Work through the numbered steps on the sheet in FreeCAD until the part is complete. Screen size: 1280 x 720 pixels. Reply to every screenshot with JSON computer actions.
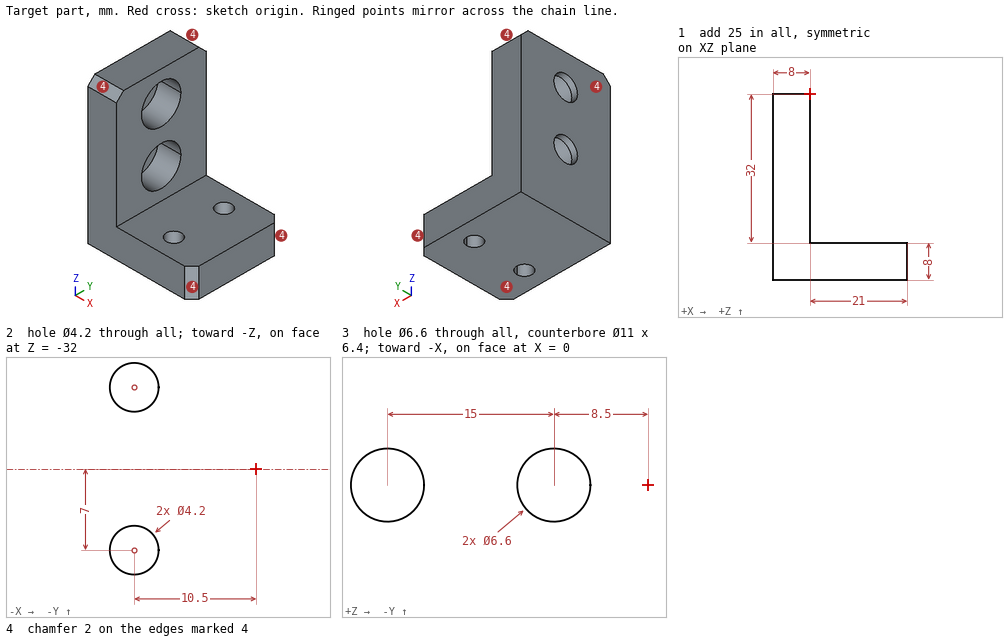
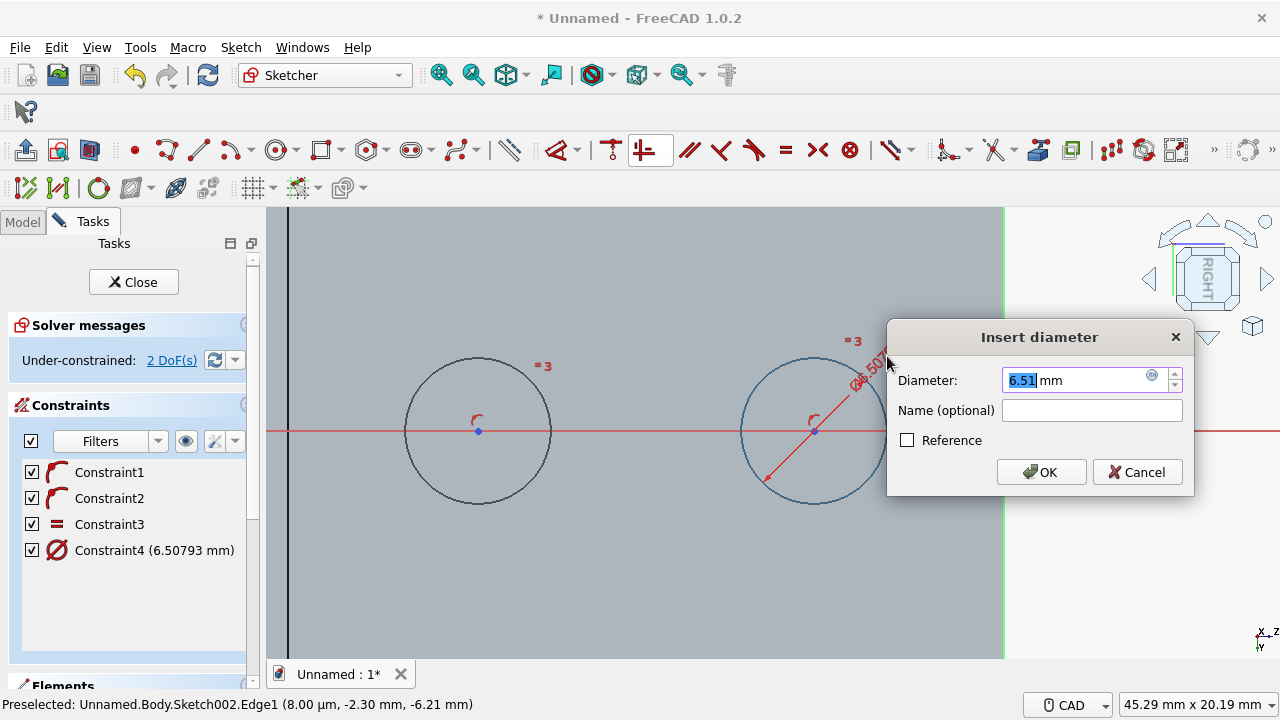
{"action": "type", "text": "6.6"}
{"action": "key", "text": "Return"}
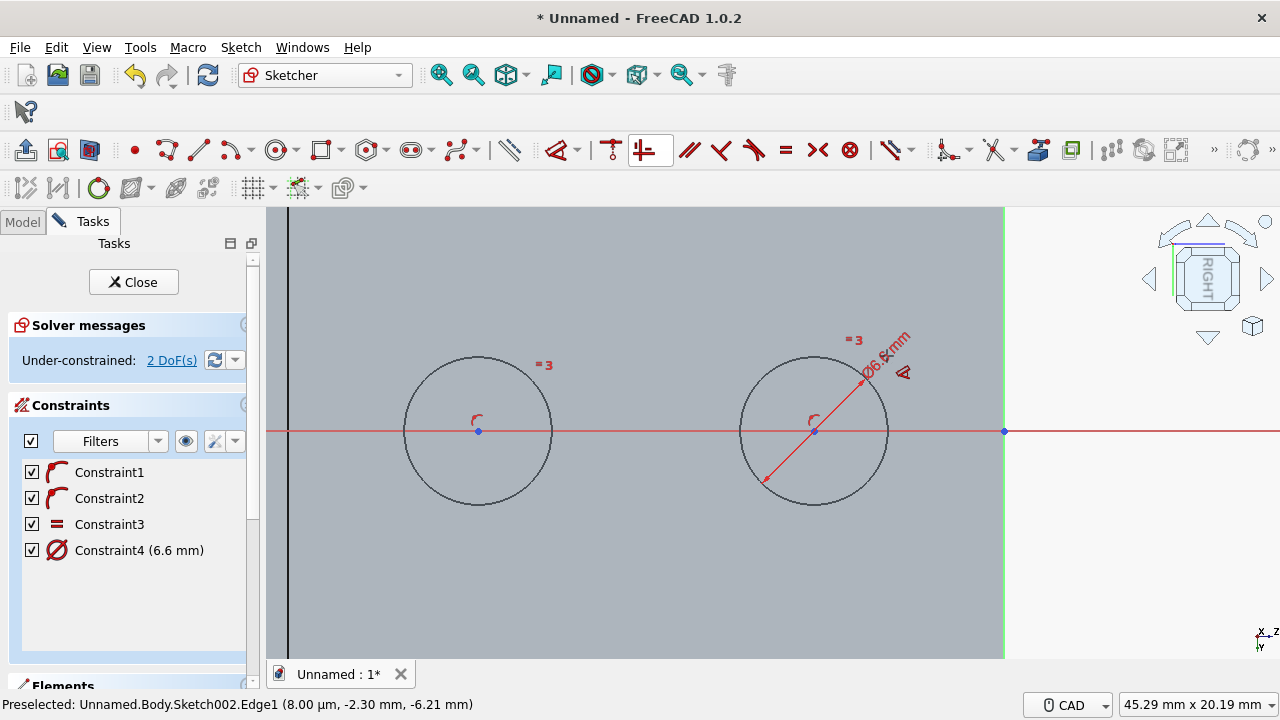
{"action": "left_click", "coordinate": [814, 431]}
{"action": "left_click", "coordinate": [909, 465]}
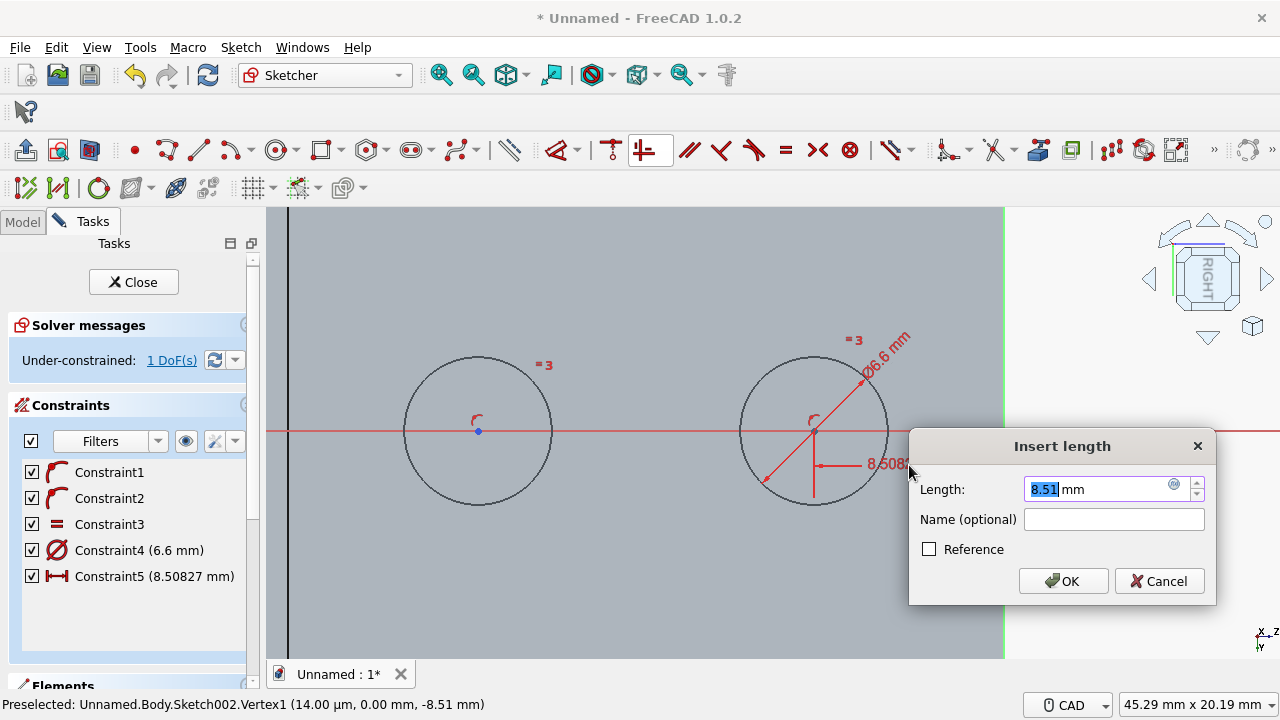
{"action": "type", "text": "8.5"}
{"action": "key", "text": "Return"}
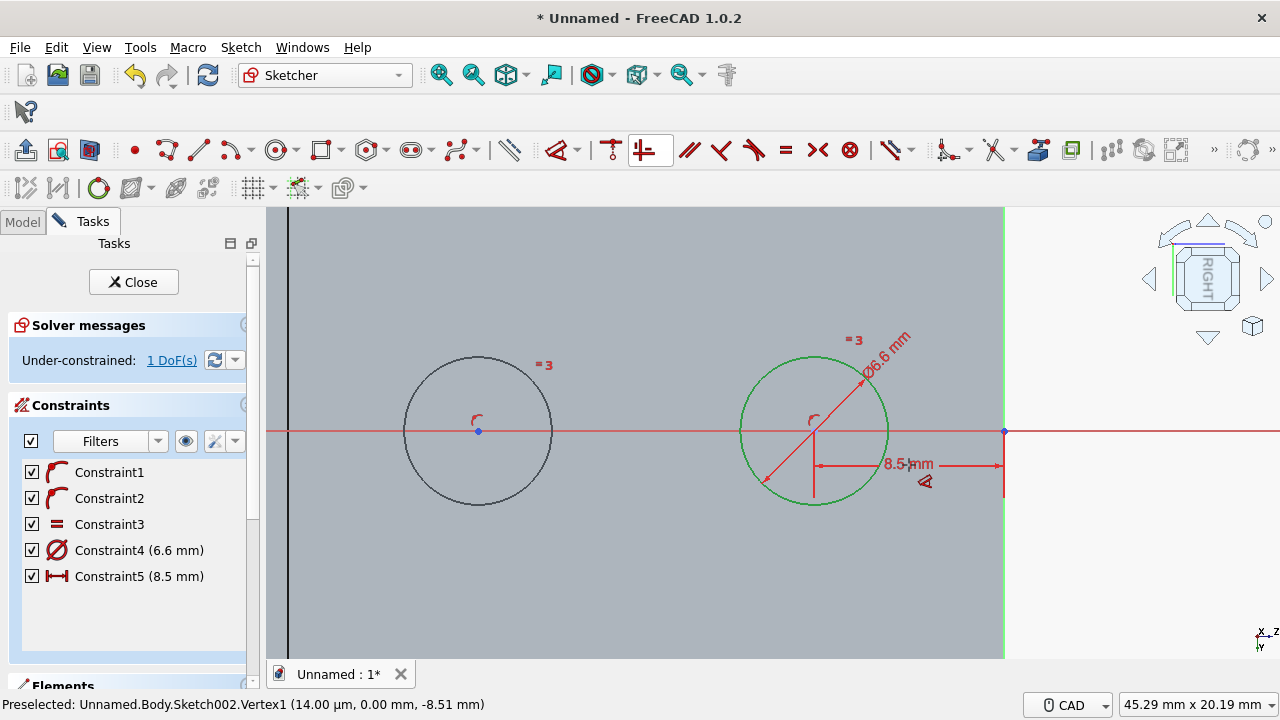
{"action": "left_click", "coordinate": [814, 431]}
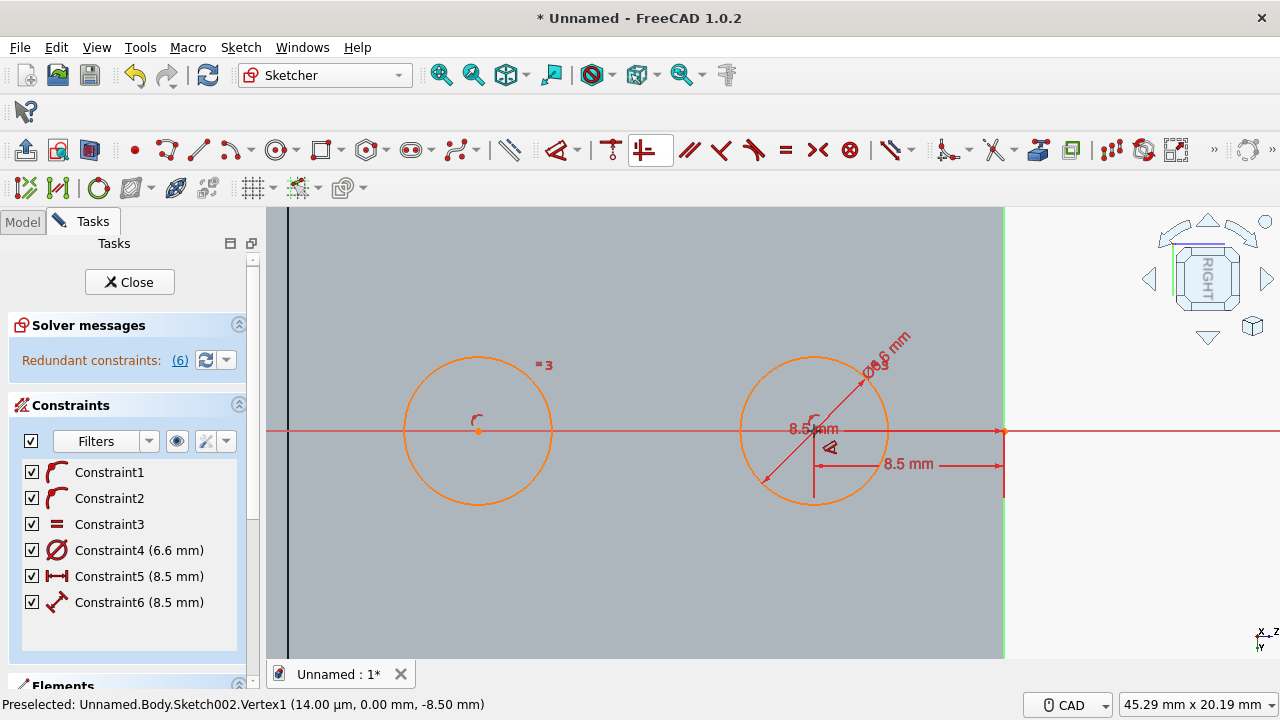
{"action": "left_click", "coordinate": [478, 431]}
{"action": "left_click", "coordinate": [646, 465]}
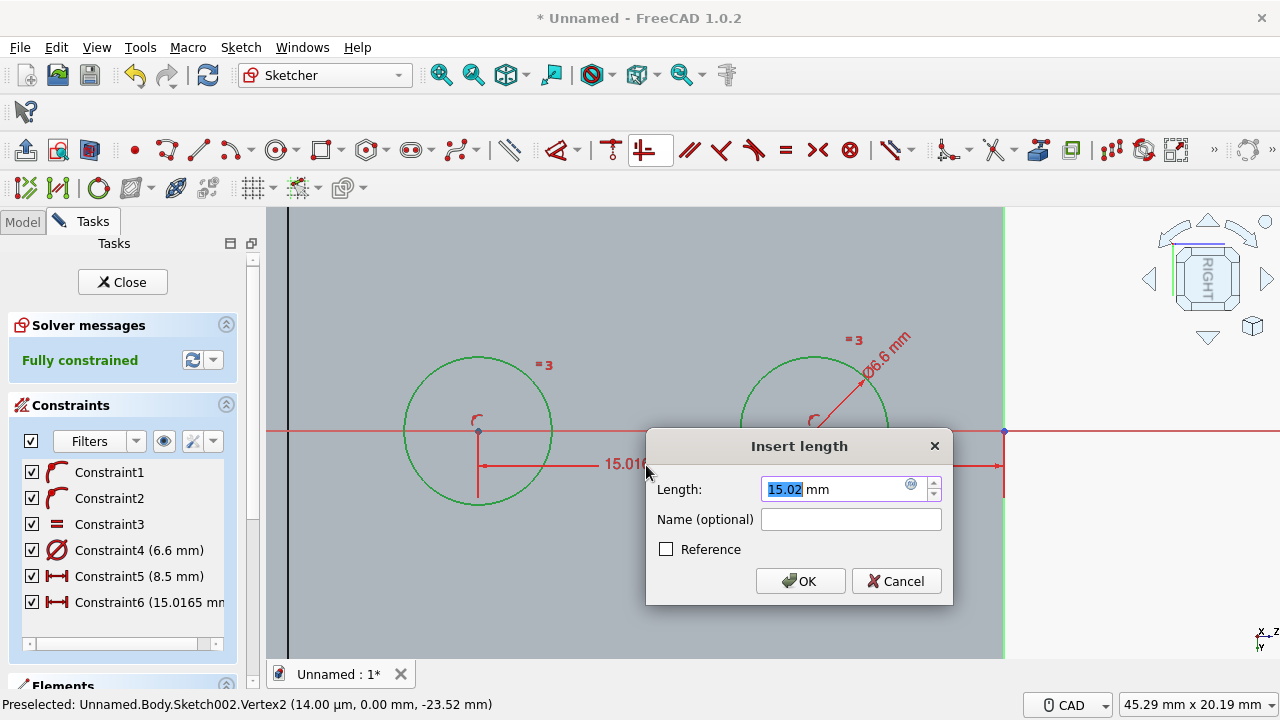
{"action": "type", "text": "15"}
{"action": "key", "text": "Return"}
{"action": "key", "text": "Escape"}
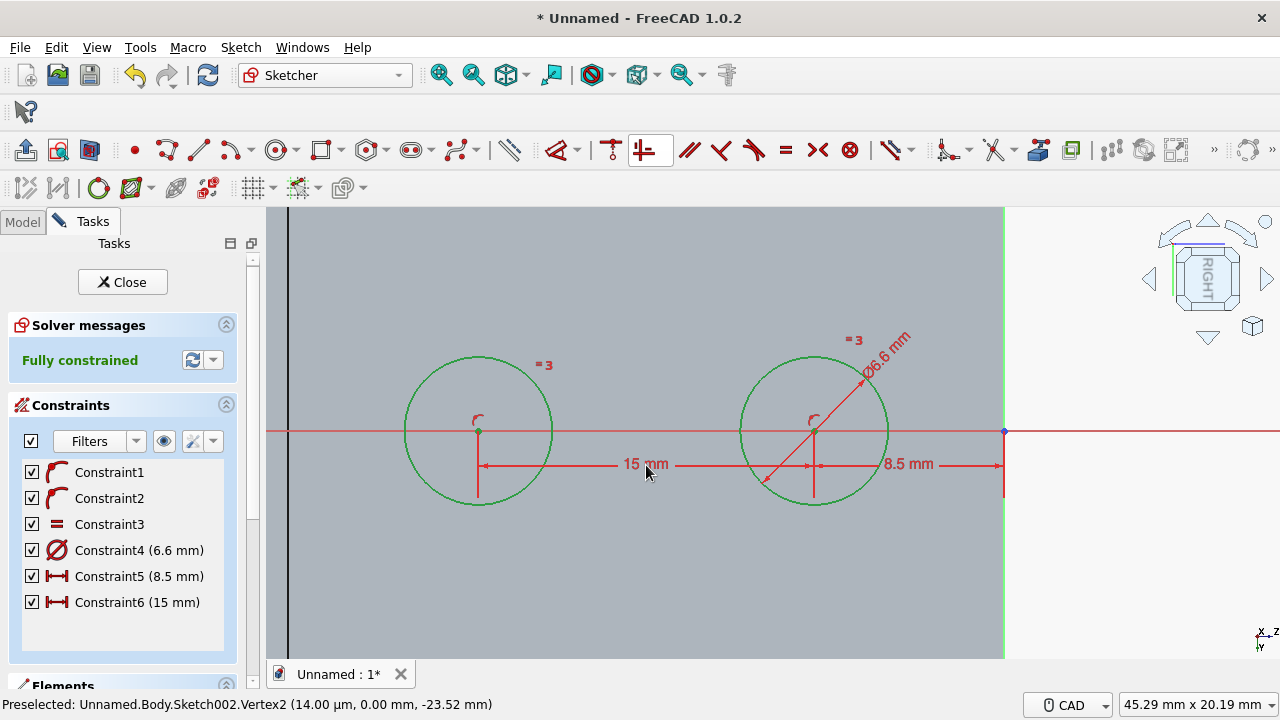
{"action": "left_click", "coordinate": [123, 282]}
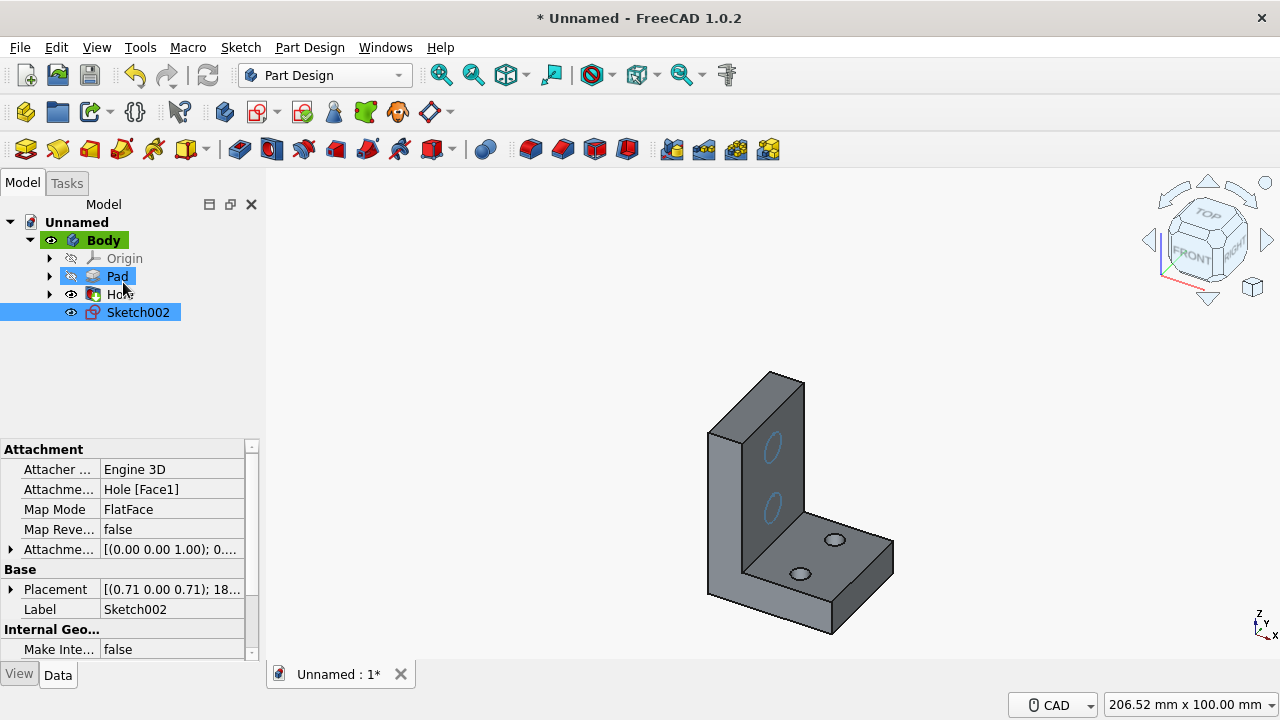
{"action": "left_click", "coordinate": [272, 150]}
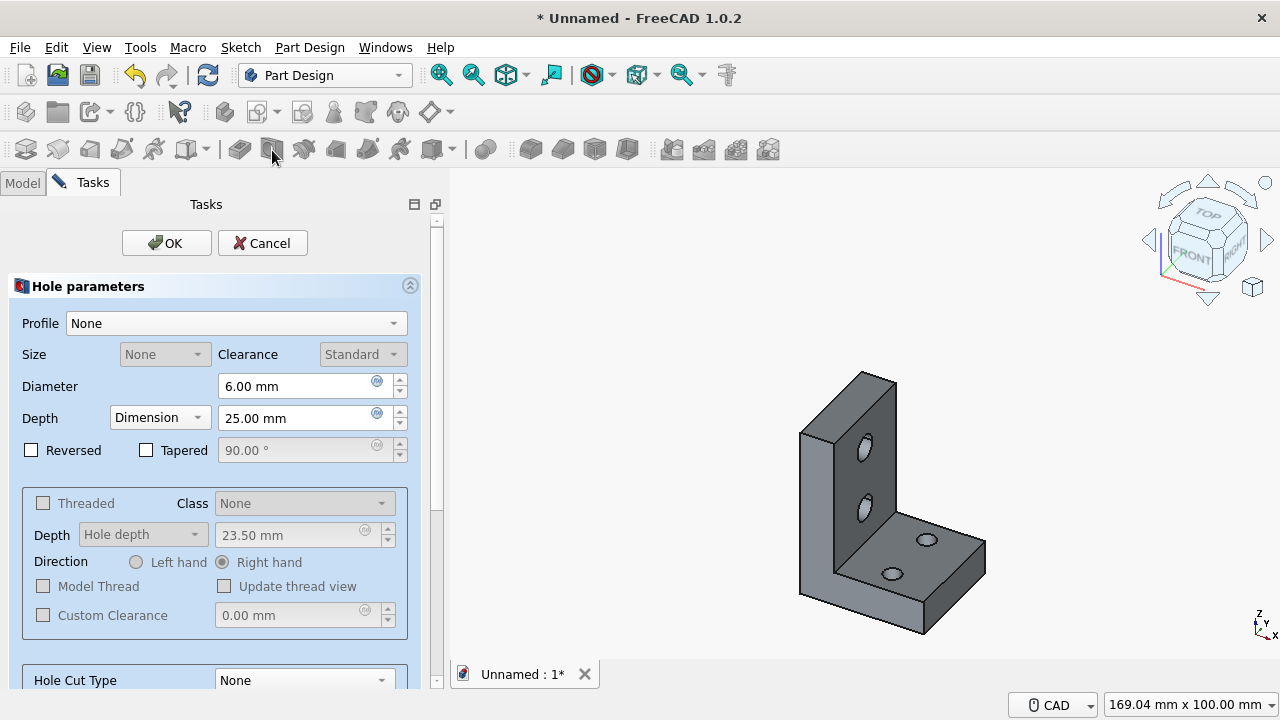
{"action": "triple_click", "coordinate": [305, 386]}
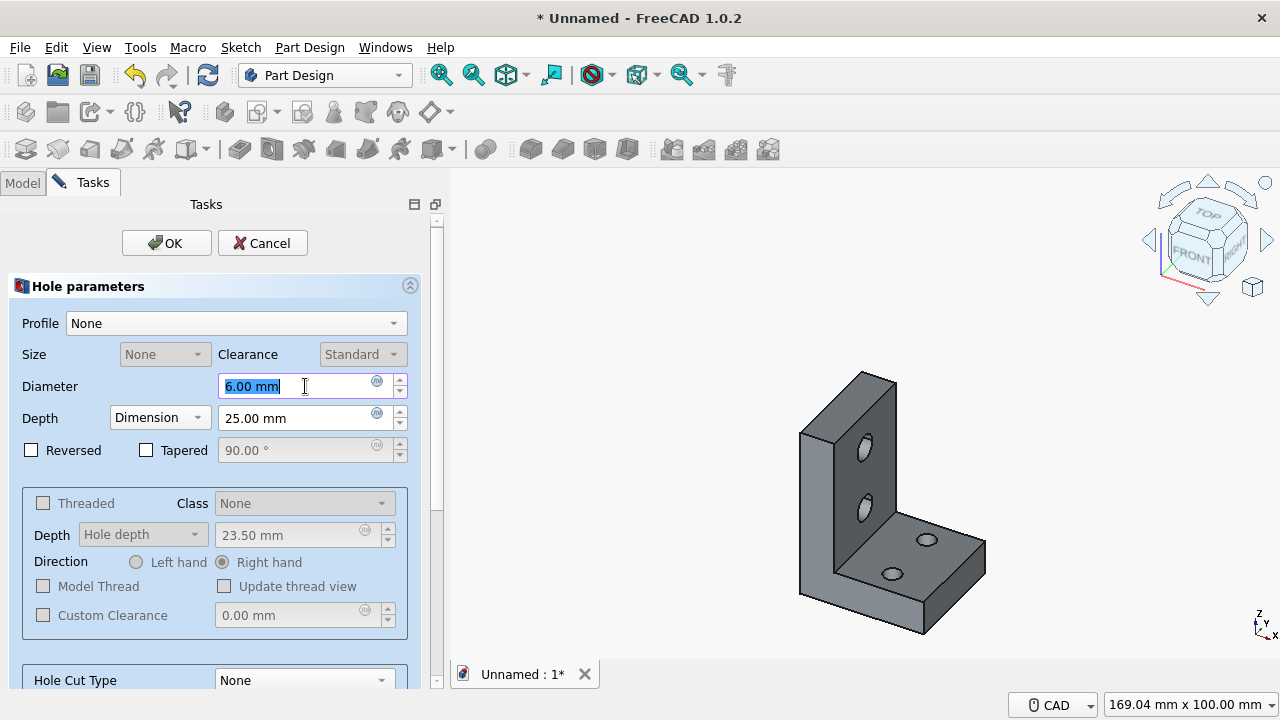
{"action": "type", "text": "6.6"}
{"action": "key", "text": "Tab"}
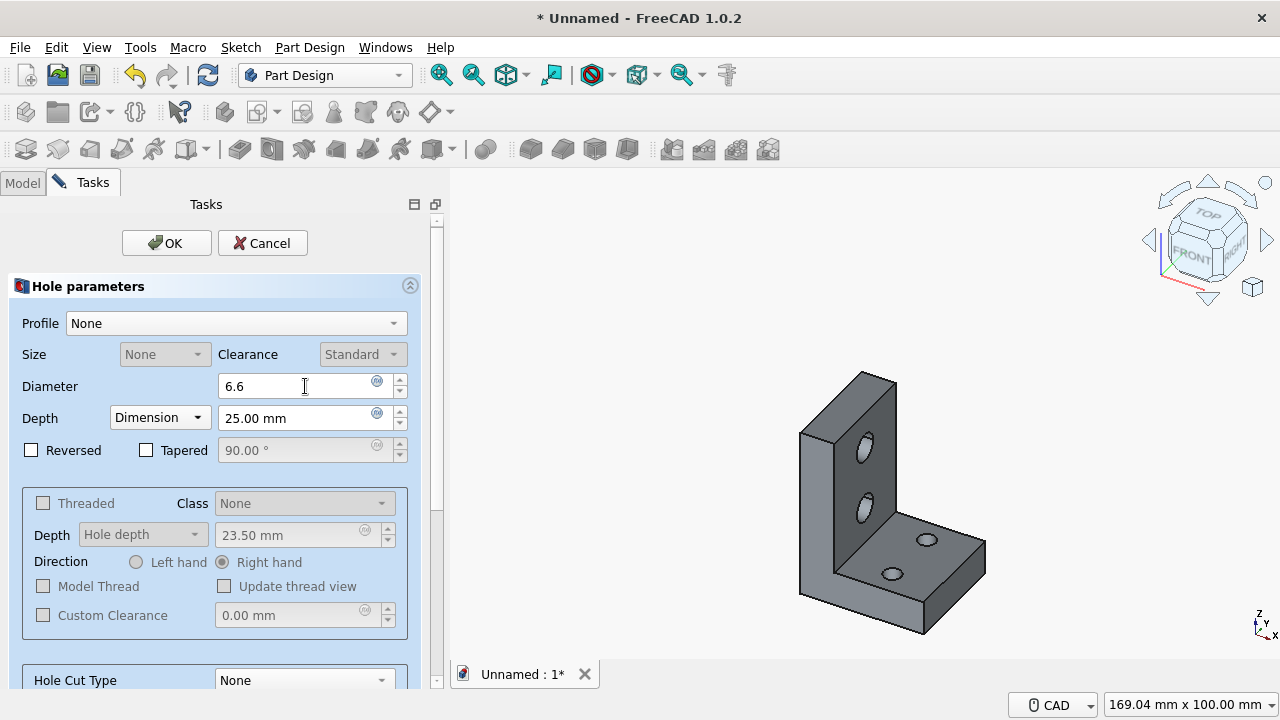
{"action": "left_click", "coordinate": [161, 418]}